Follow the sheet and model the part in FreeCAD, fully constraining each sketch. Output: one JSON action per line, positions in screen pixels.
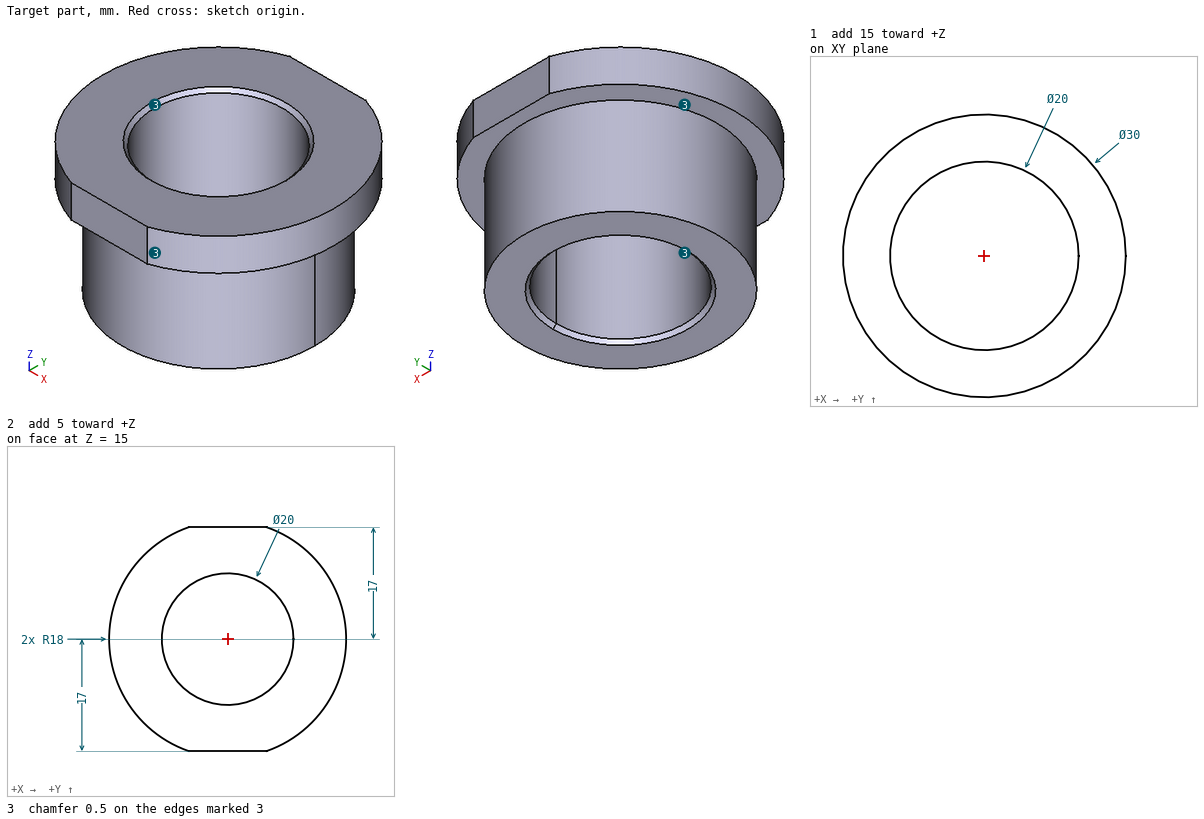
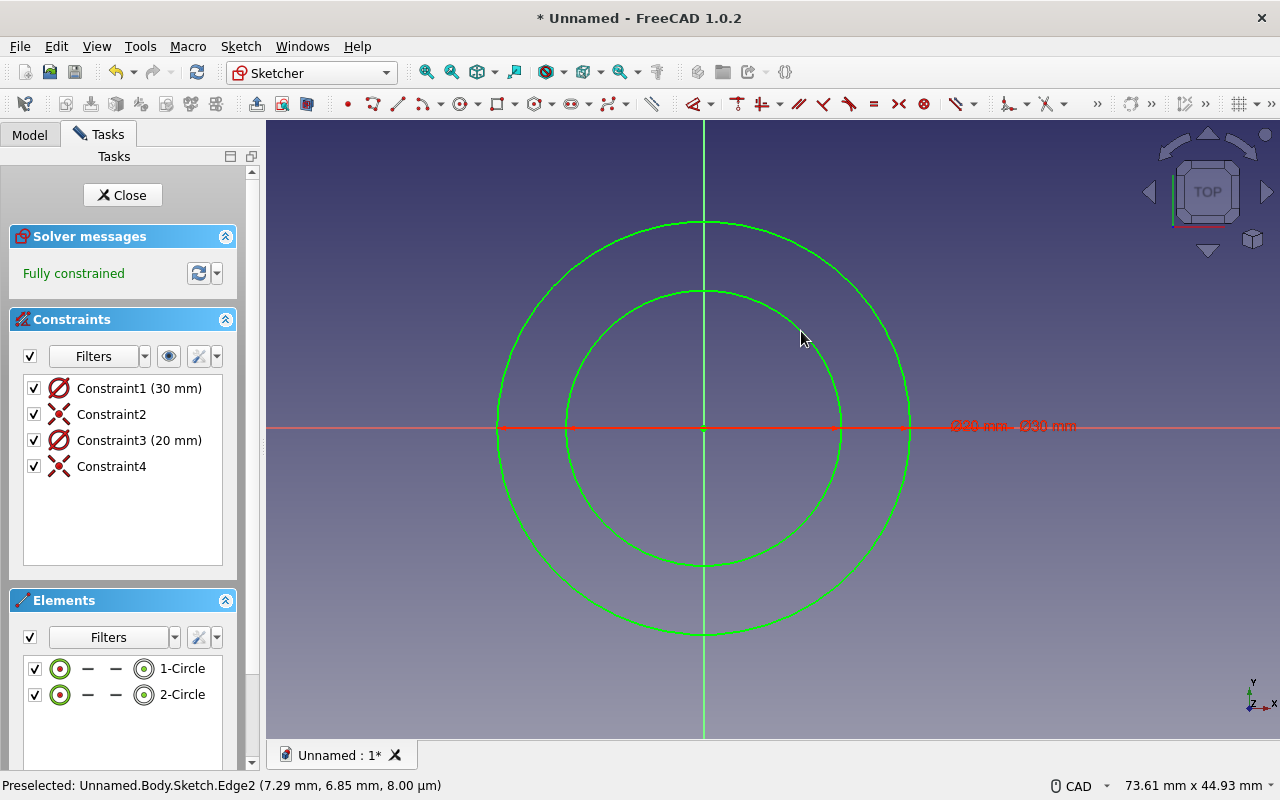
{"action": "left_click", "coordinate": [123, 195]}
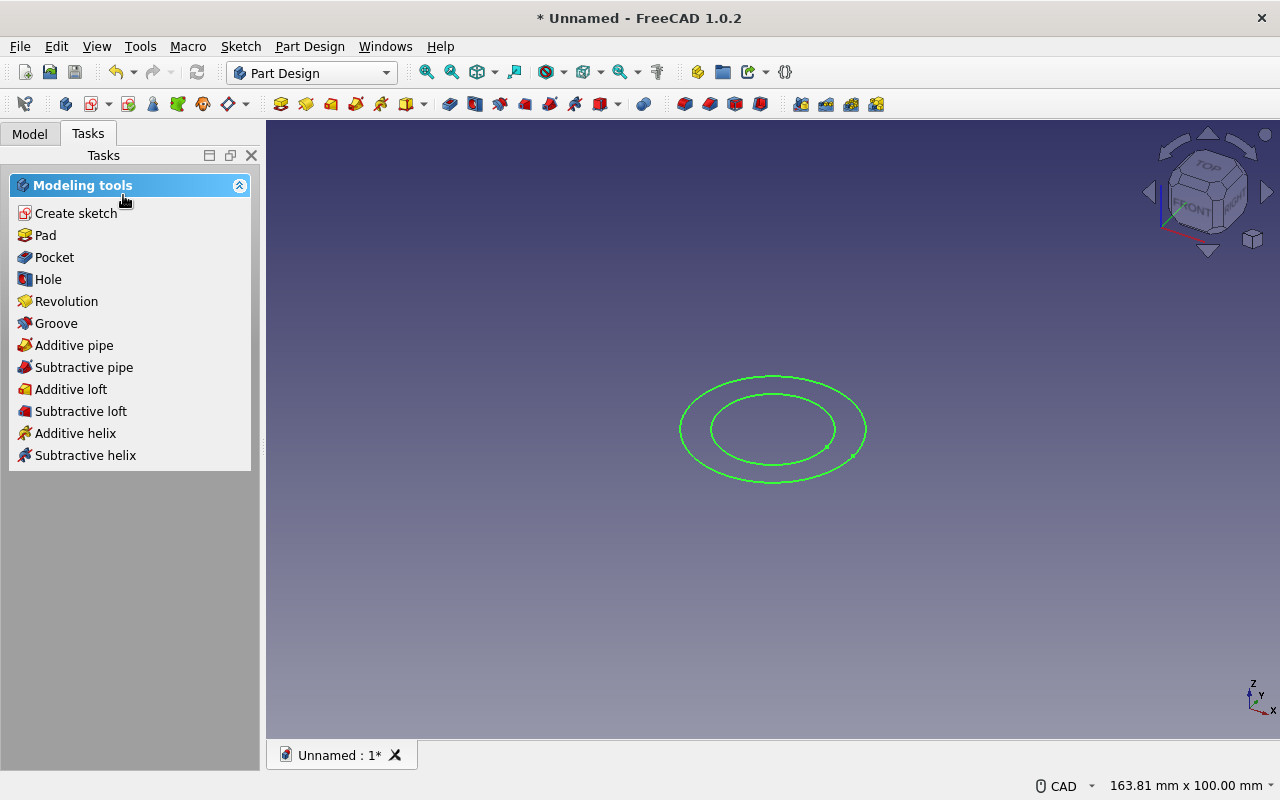
{"action": "left_click", "coordinate": [281, 104]}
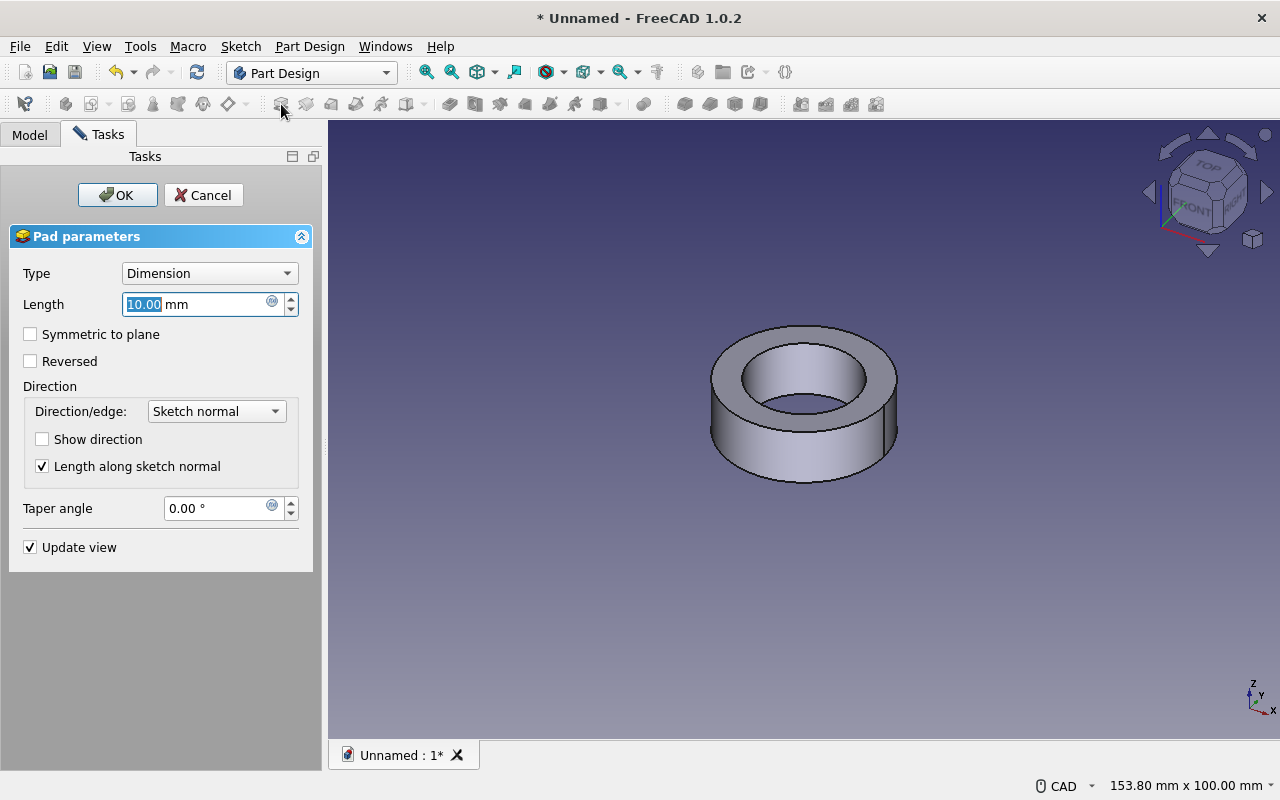
{"action": "type", "text": "15"}
{"action": "key", "text": "Tab"}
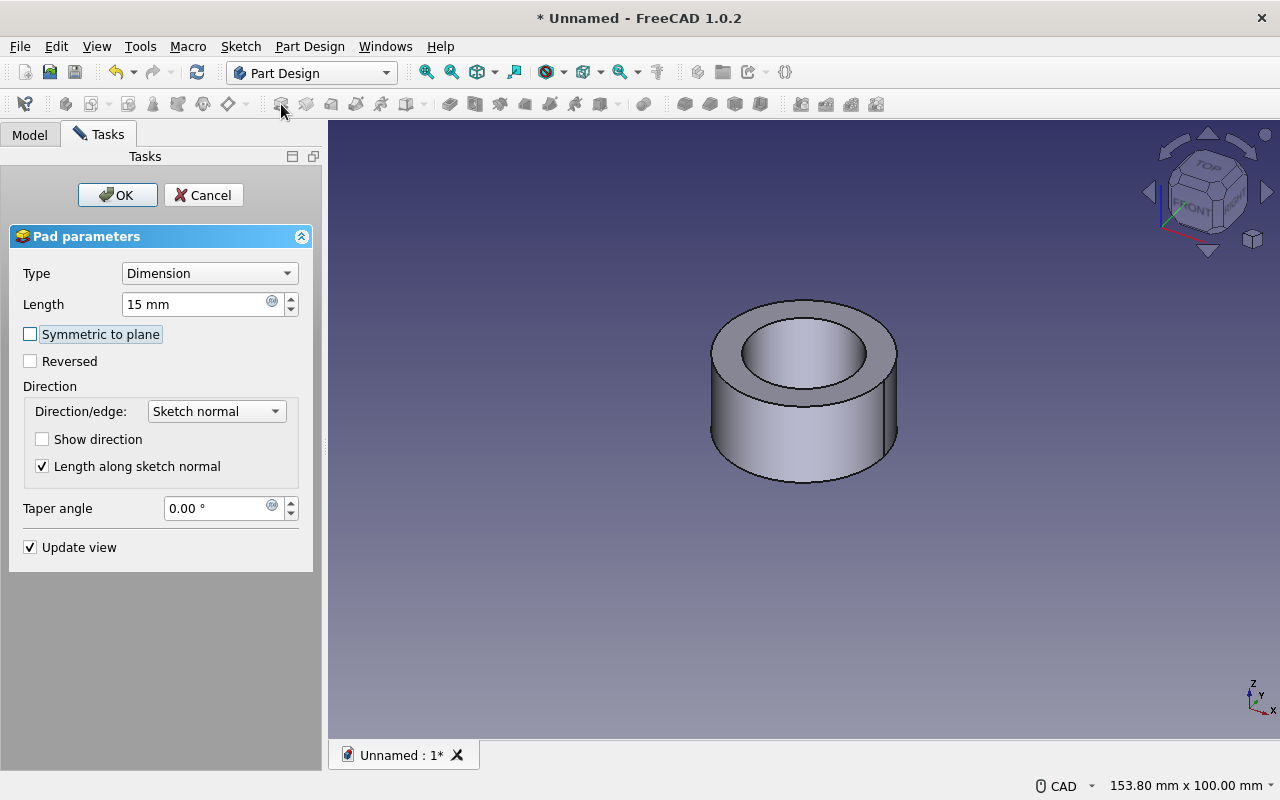
{"action": "left_click", "coordinate": [118, 195]}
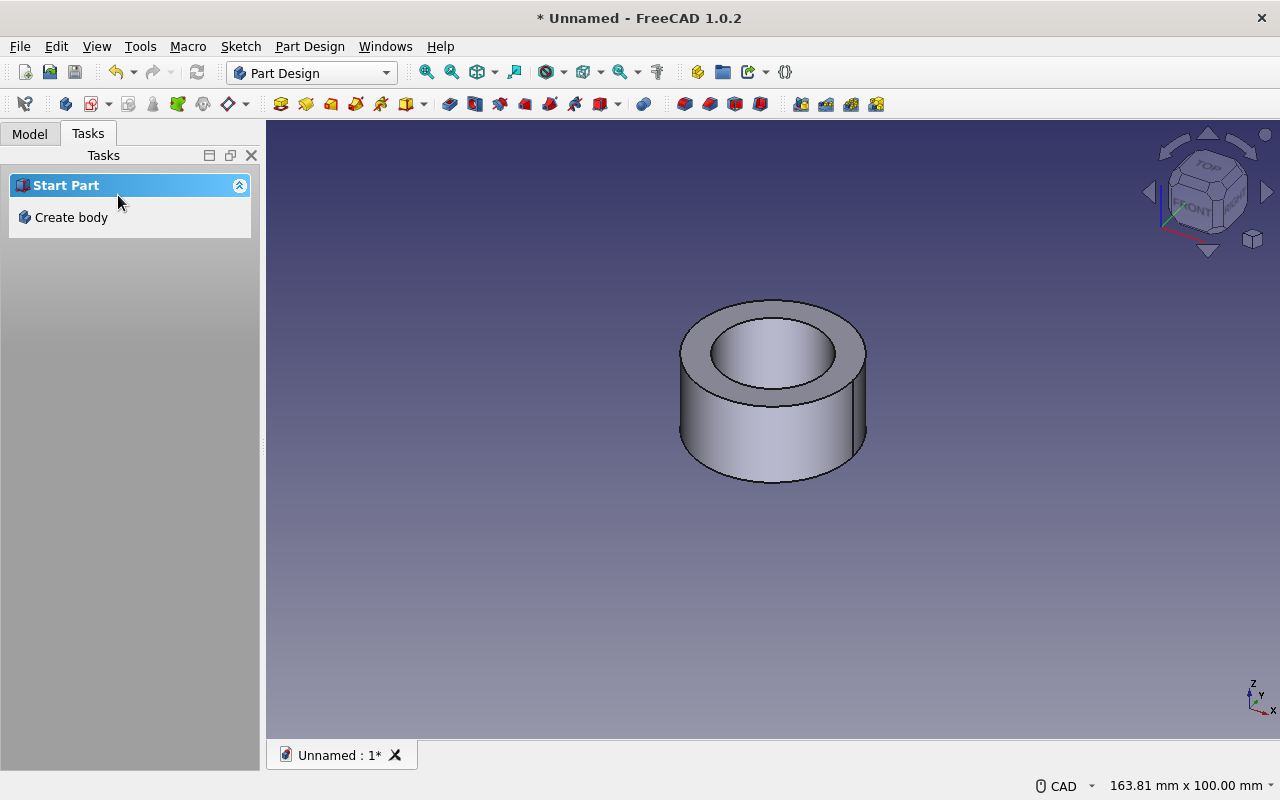
{"action": "left_click", "coordinate": [427, 72]}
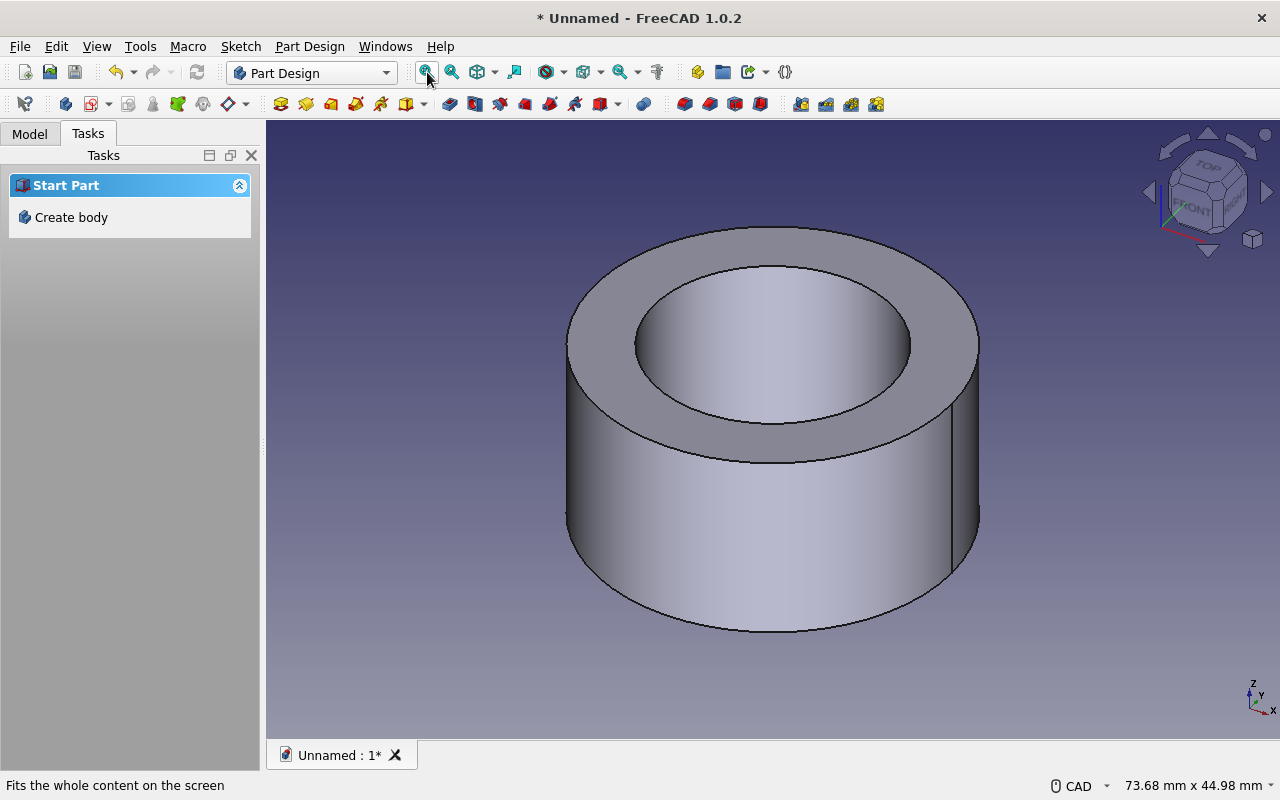
{"action": "left_click", "coordinate": [926, 395]}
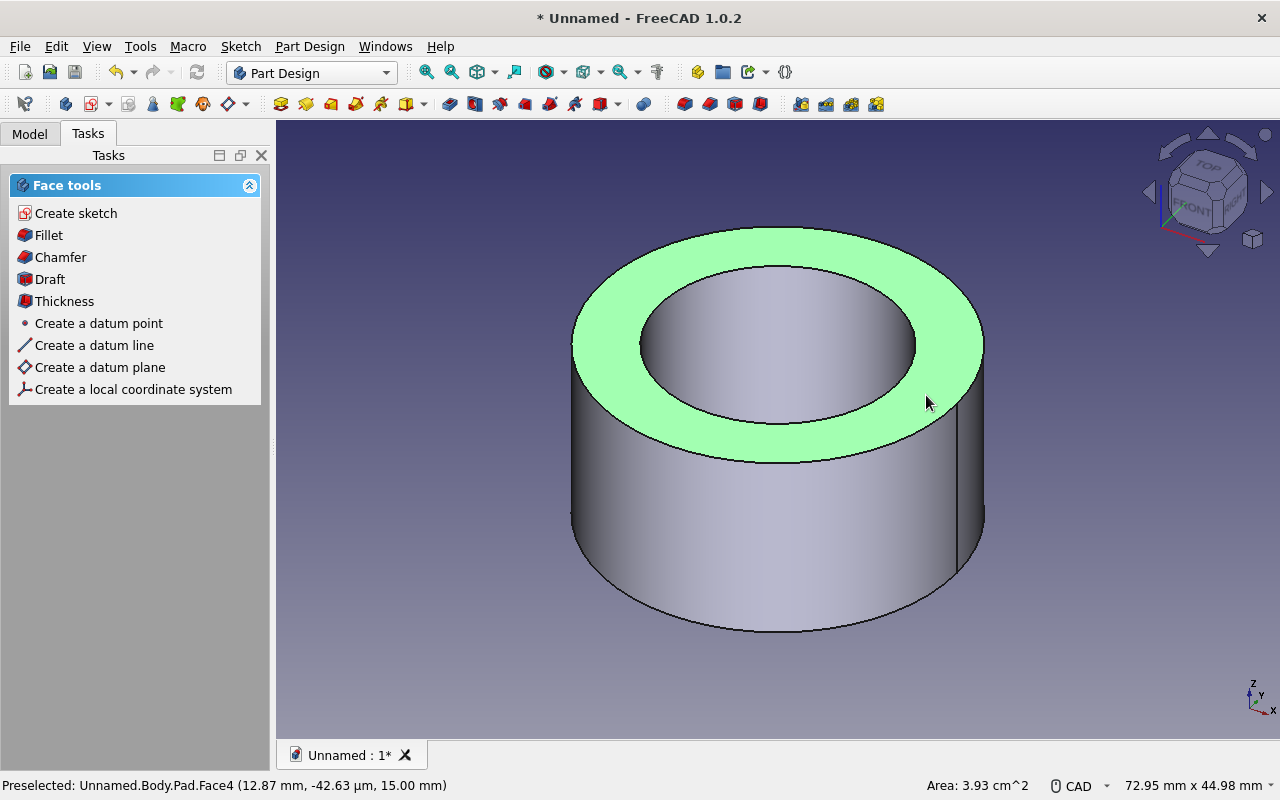
{"action": "left_click", "coordinate": [90, 104]}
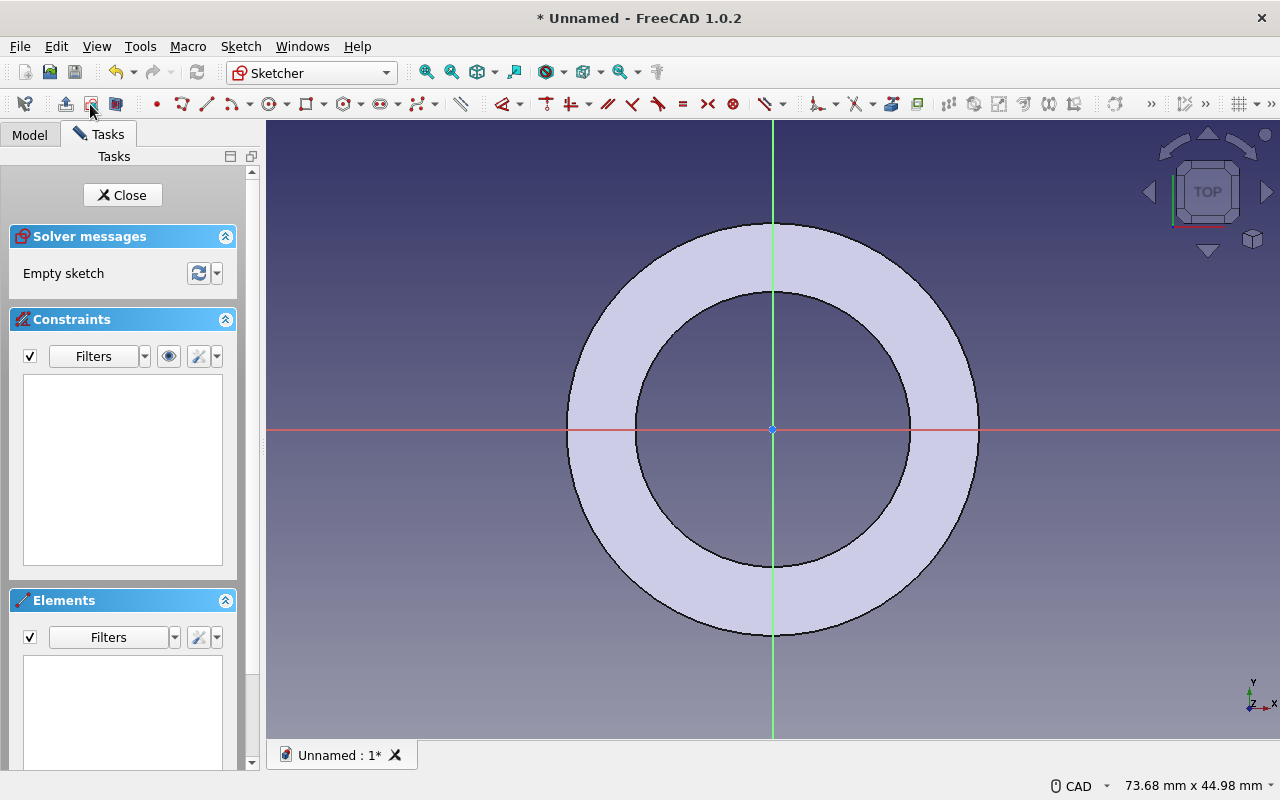
{"action": "left_click", "coordinate": [207, 104]}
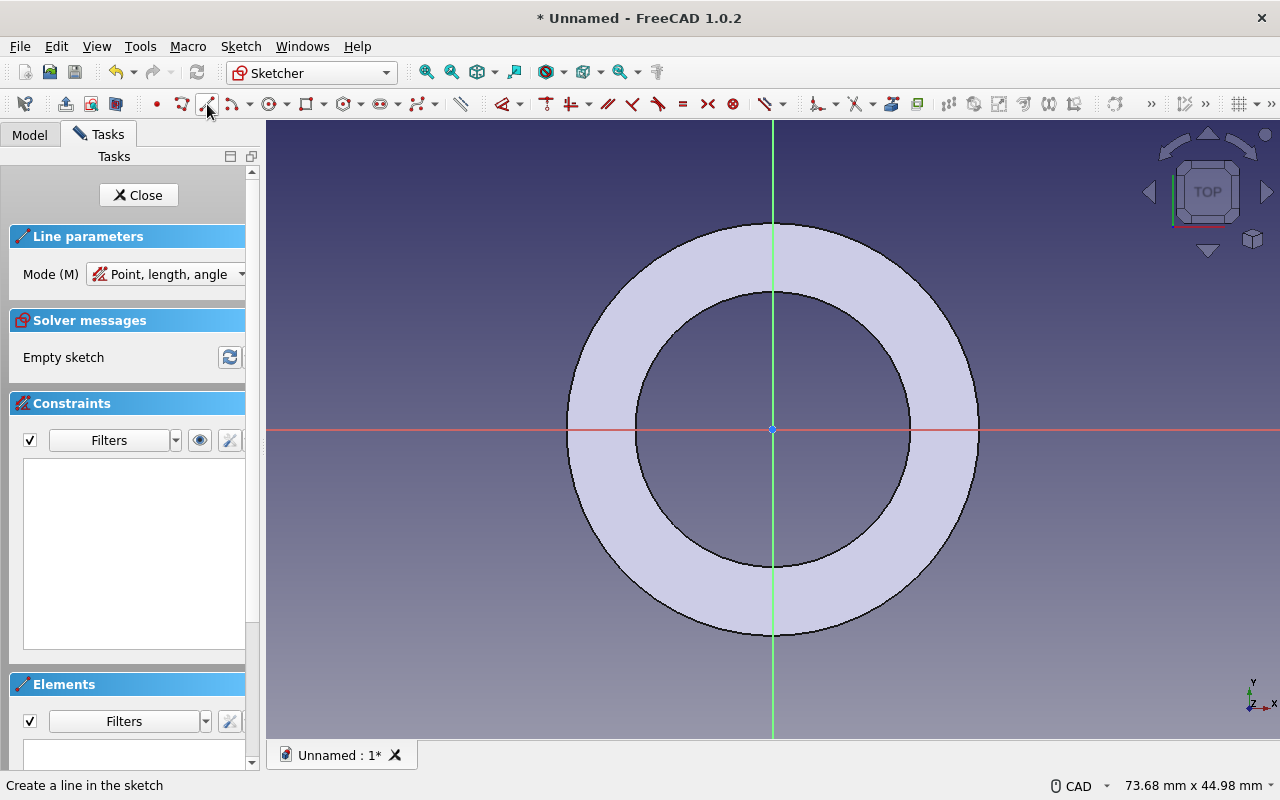
{"action": "left_click", "coordinate": [854, 196]}
{"action": "left_click", "coordinate": [691, 196]}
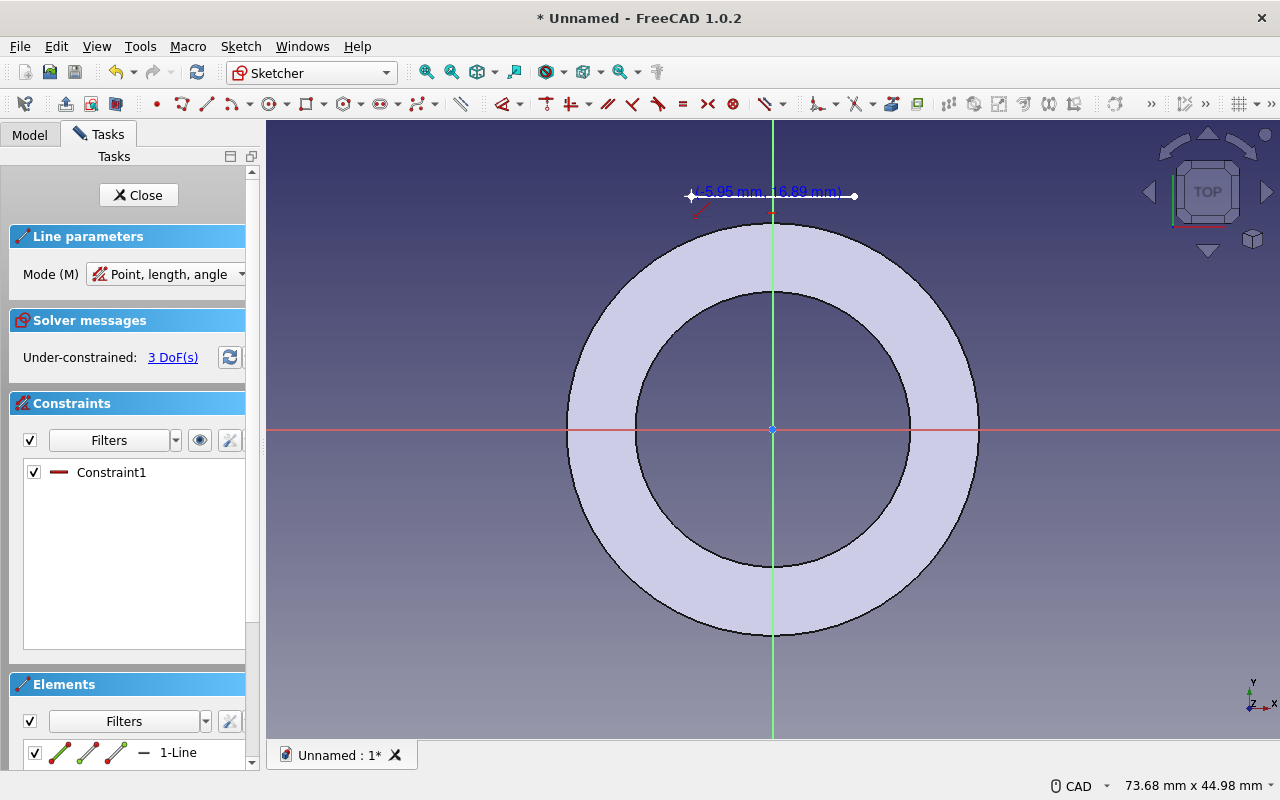
{"action": "left_click", "coordinate": [691, 663]}
{"action": "left_click", "coordinate": [854, 663]}